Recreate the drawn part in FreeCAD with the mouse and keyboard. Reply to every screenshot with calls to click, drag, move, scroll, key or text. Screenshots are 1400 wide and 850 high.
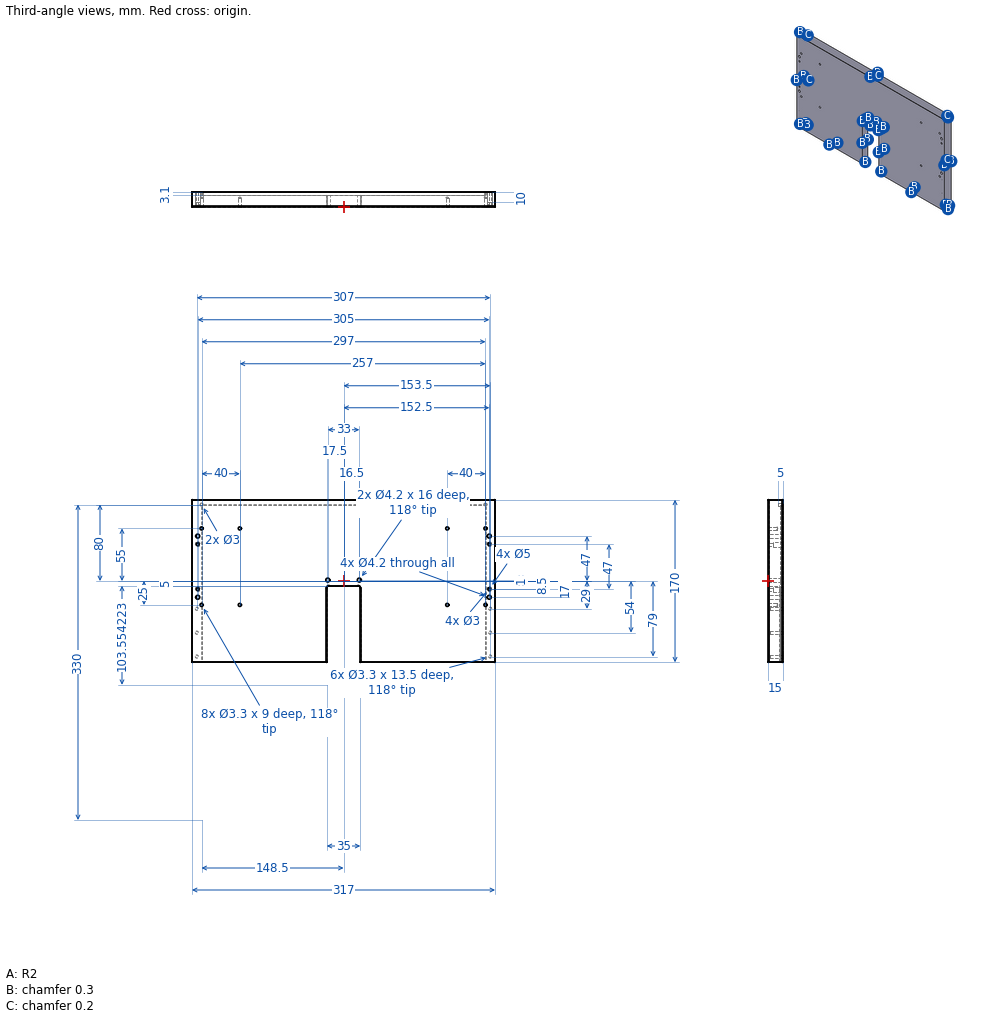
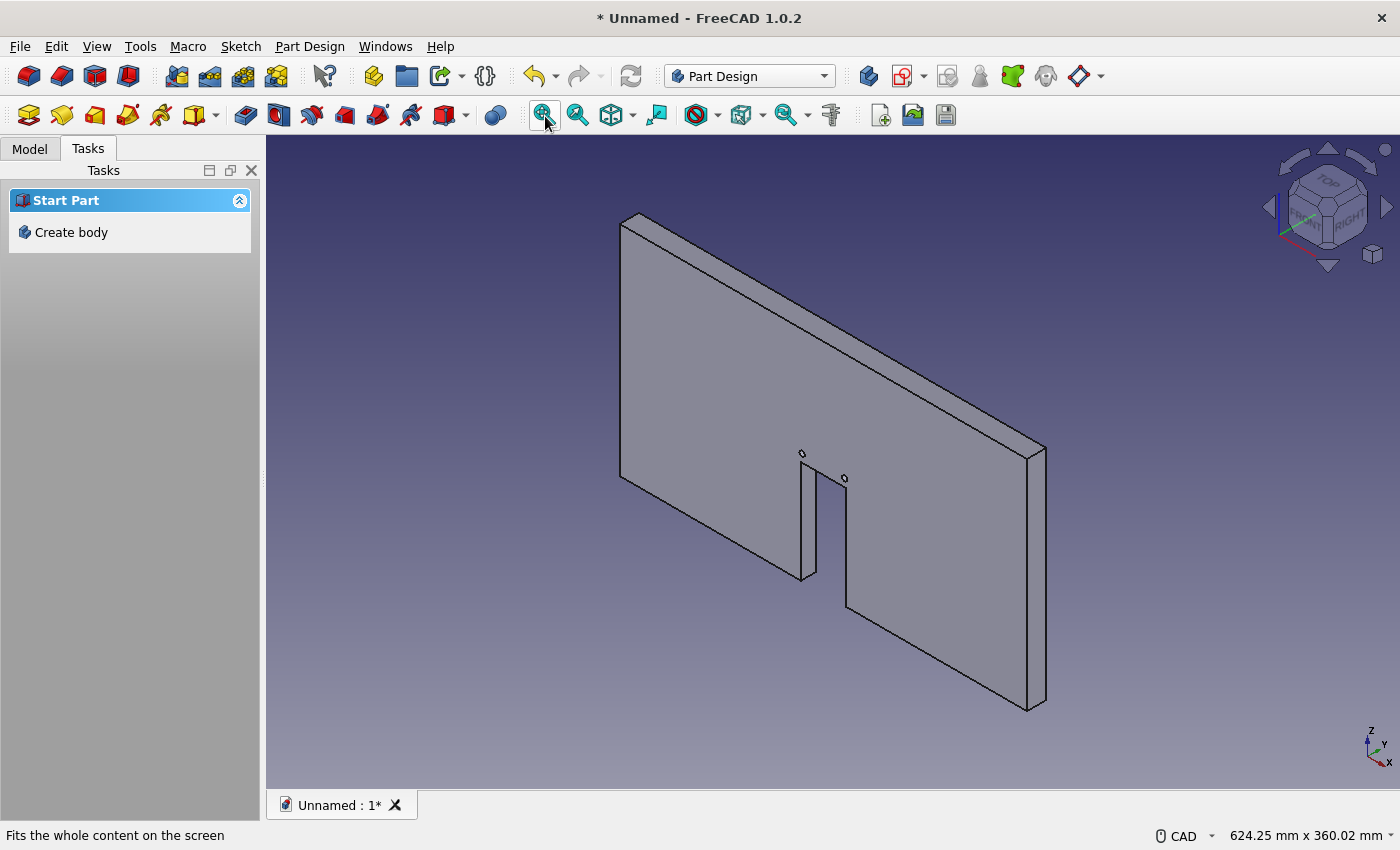
scroll(853, 483, up, 4)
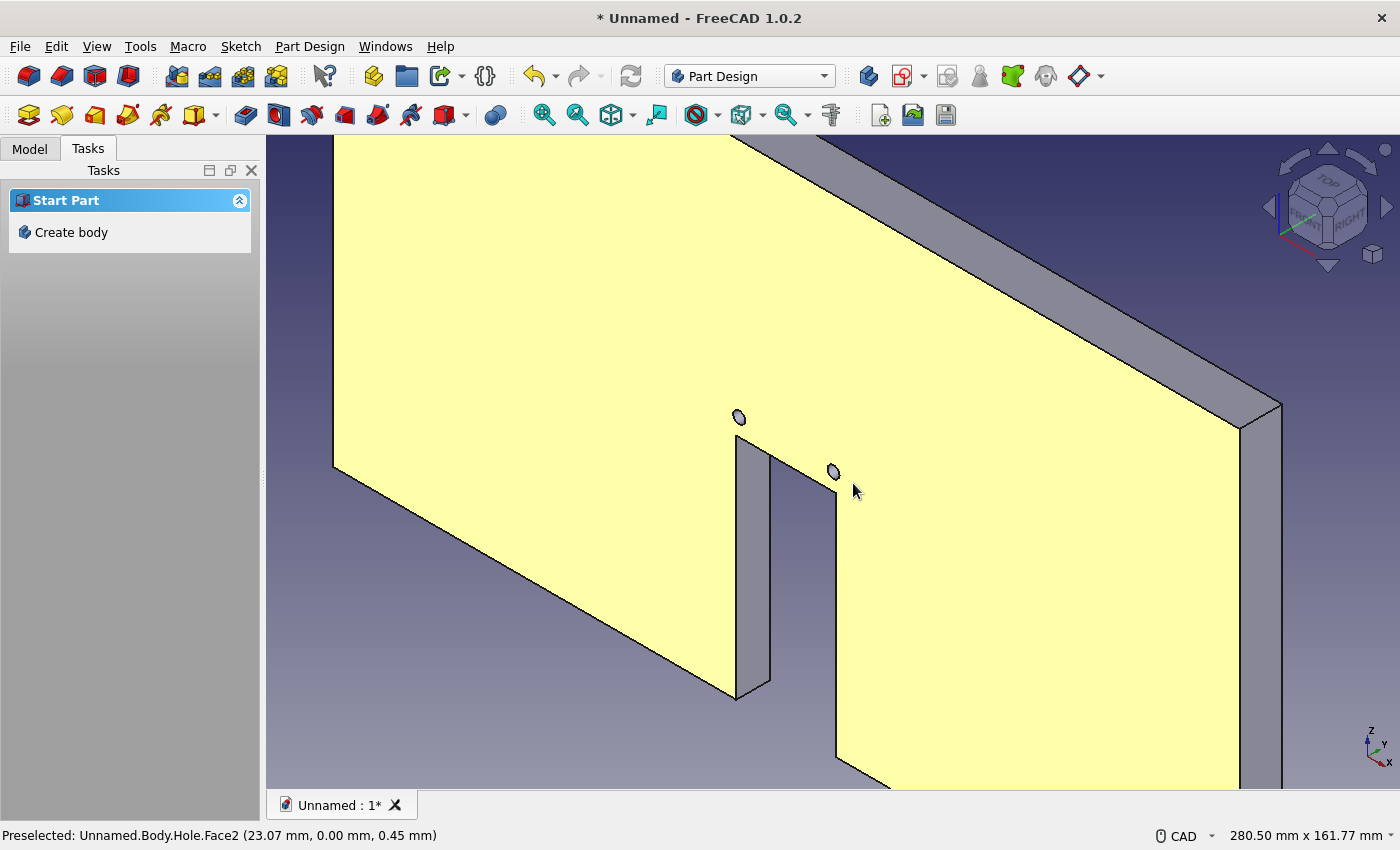
key(v)
key(f)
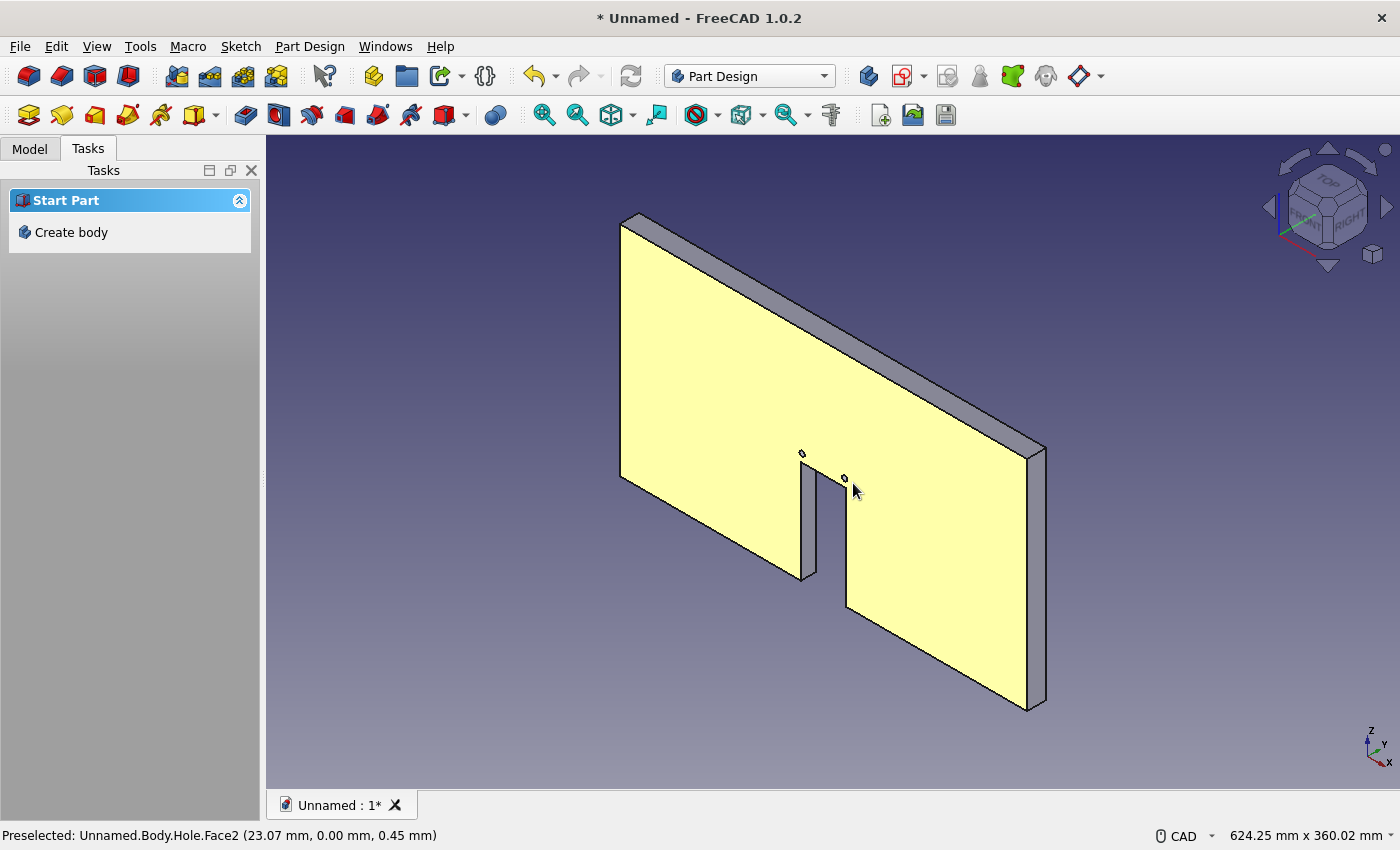
key(1)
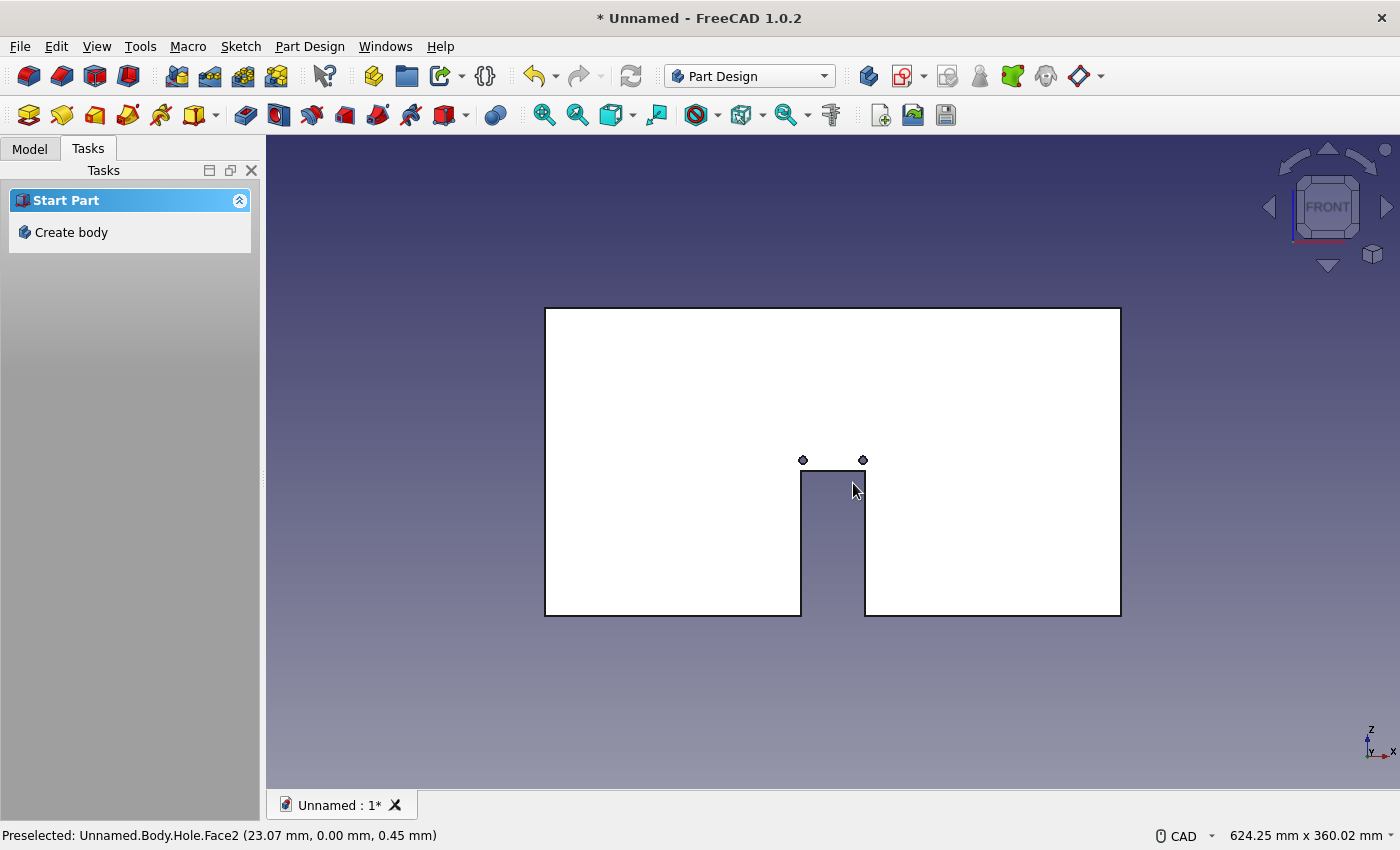
scroll(865, 470, up, 4)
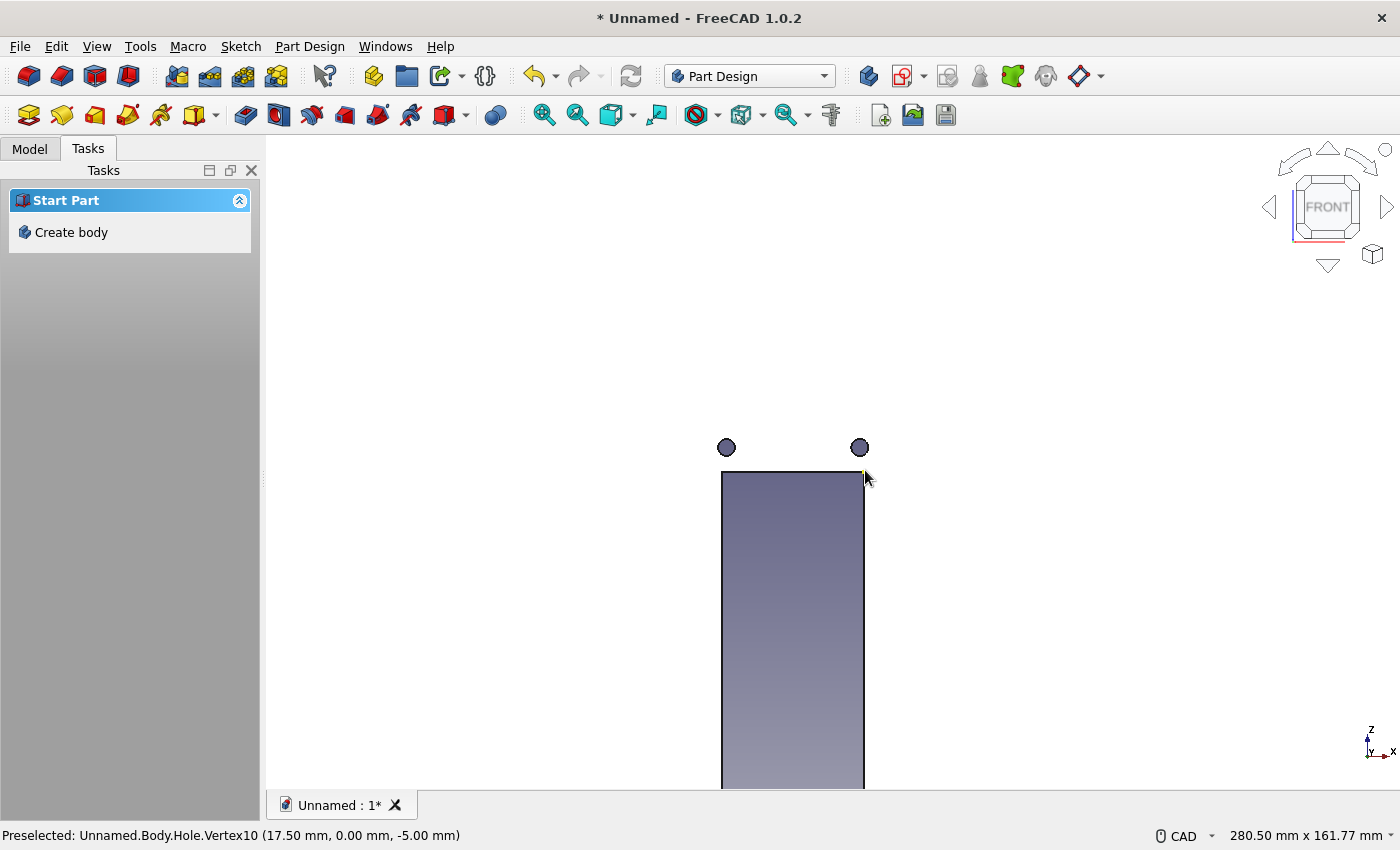
click(545, 116)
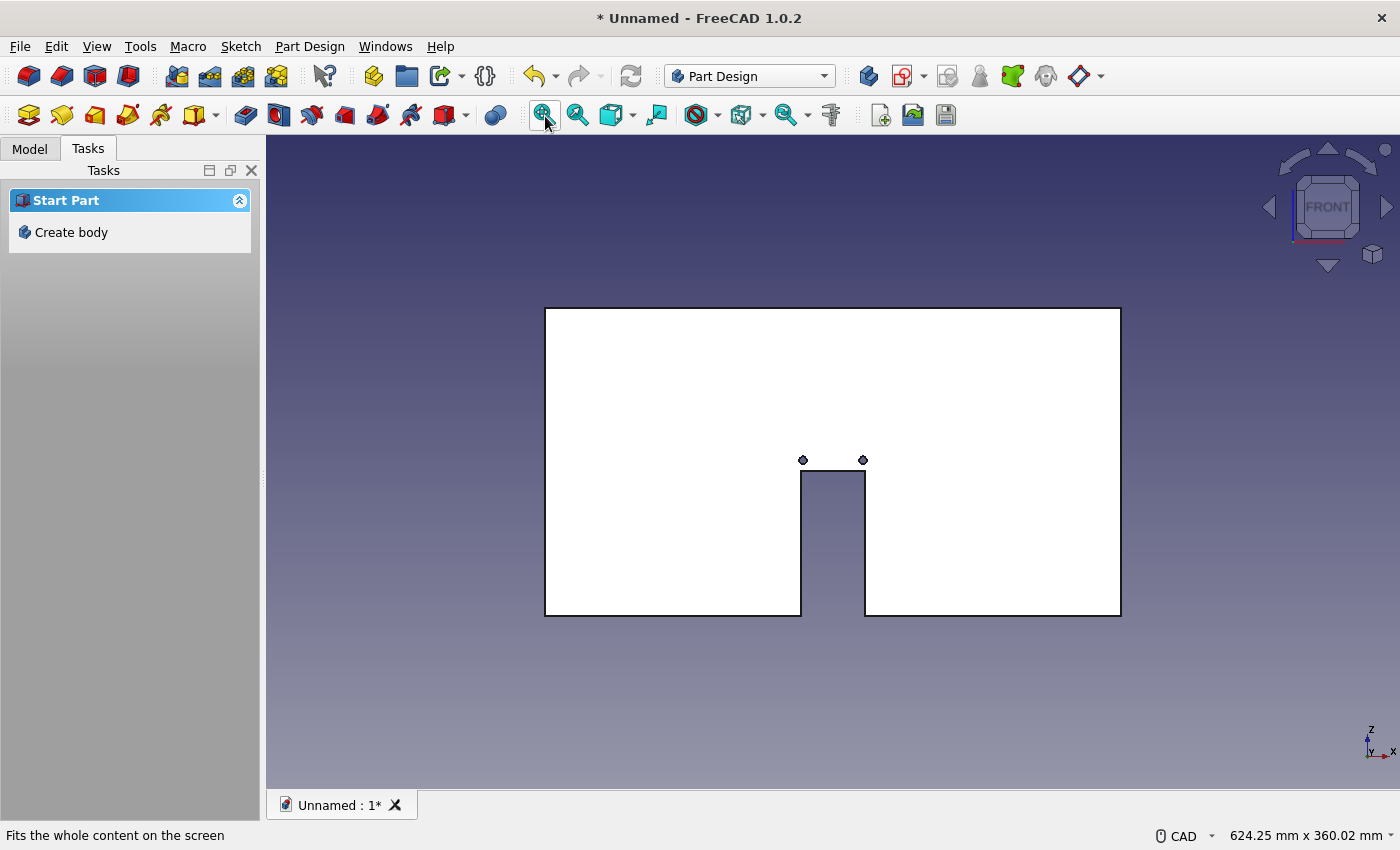
key(3)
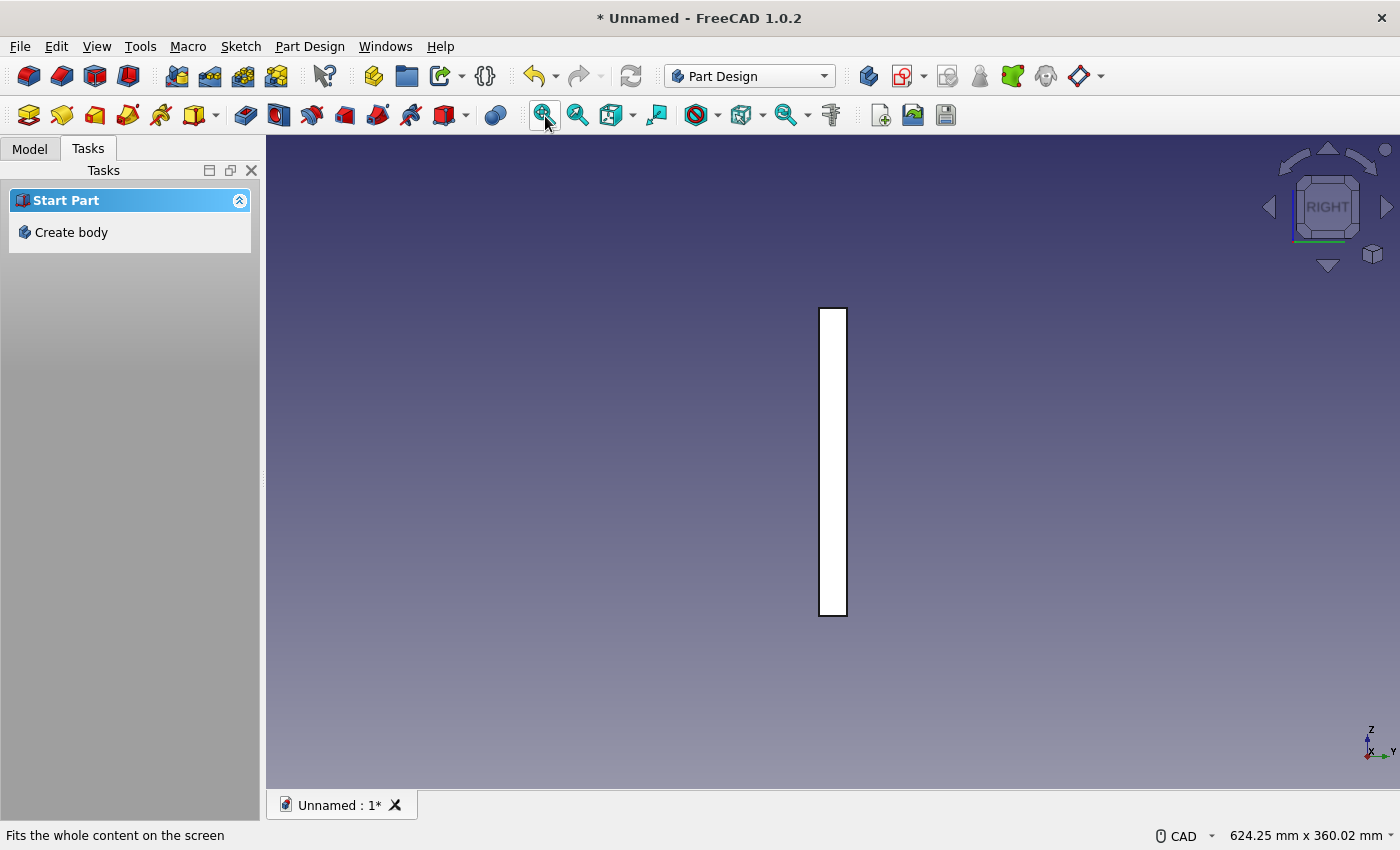
scroll(830, 470, up, 4)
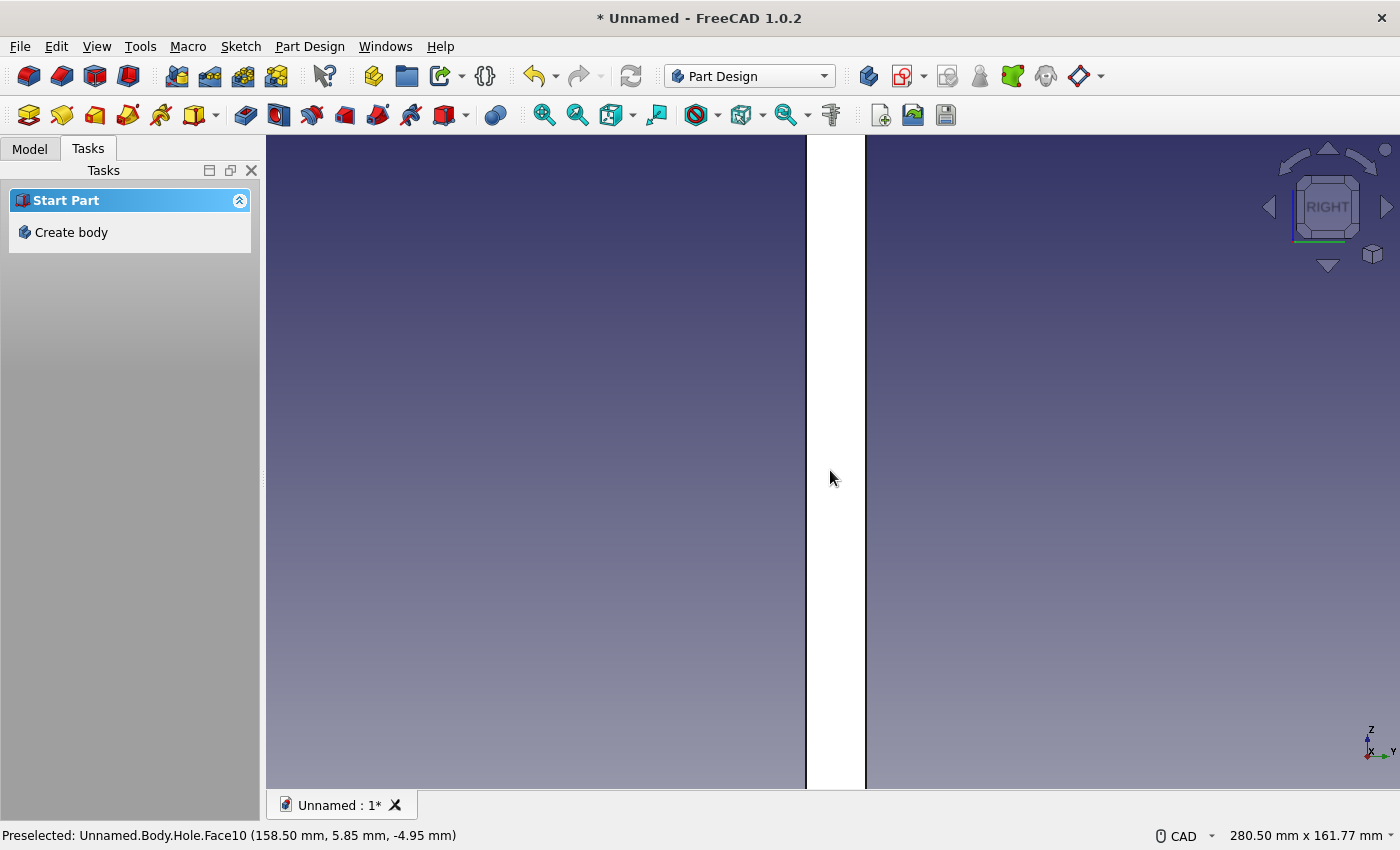
key(v)
key(f)